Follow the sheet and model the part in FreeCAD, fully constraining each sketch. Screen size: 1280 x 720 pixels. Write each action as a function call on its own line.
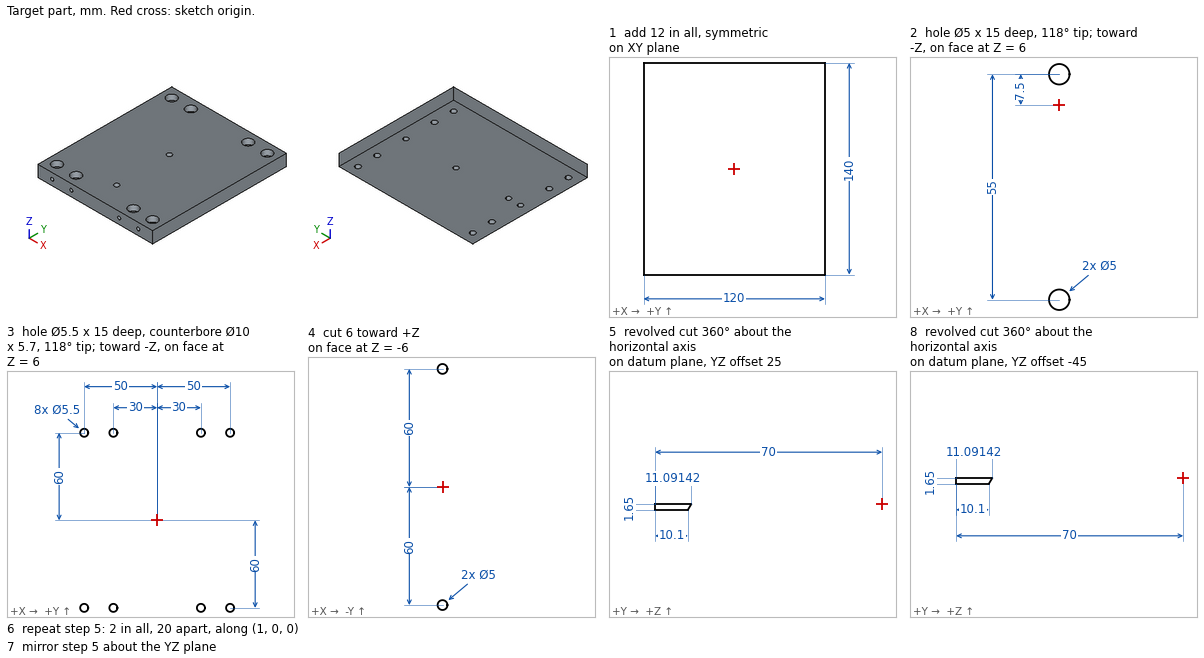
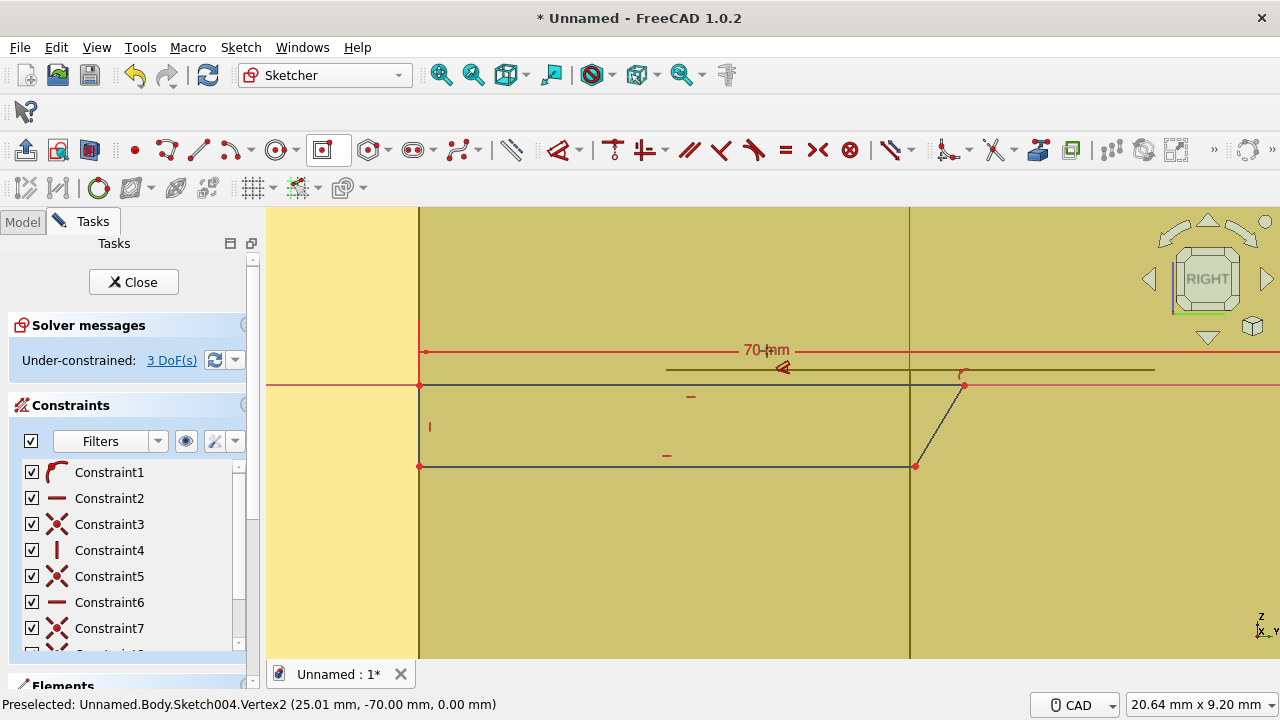
click(419, 410)
click(385, 426)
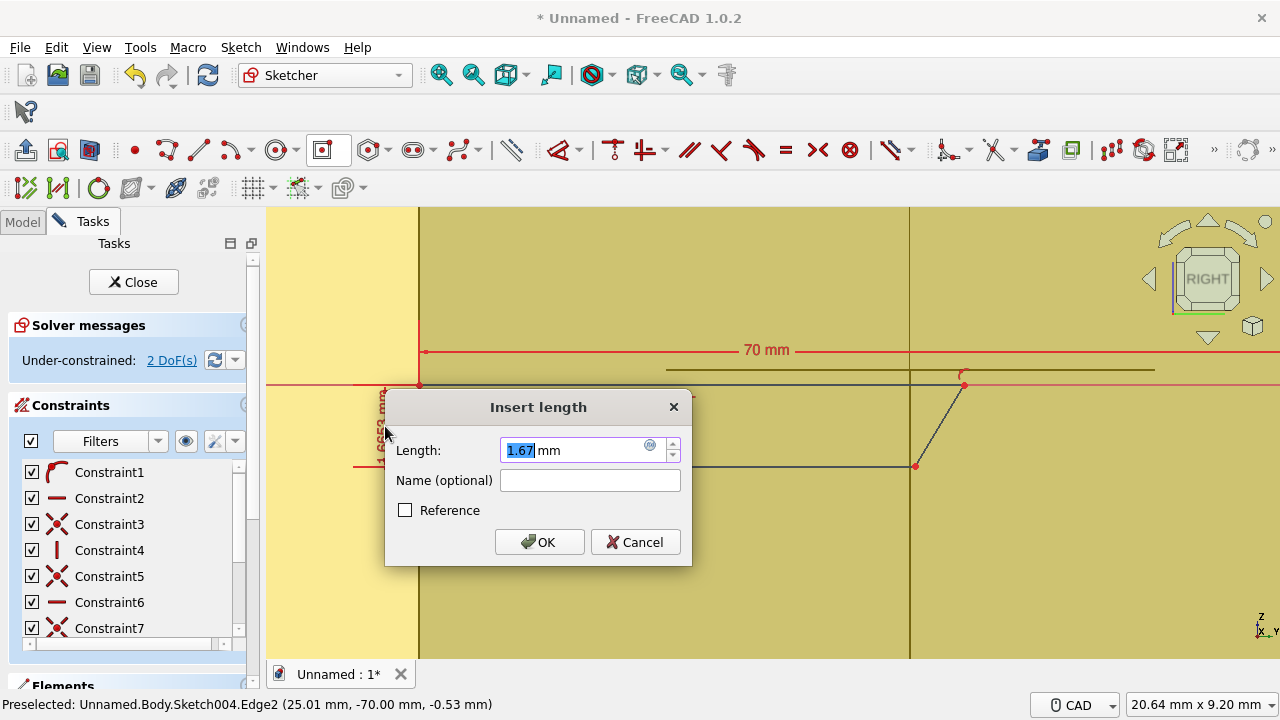
text(1.65)
key(Return)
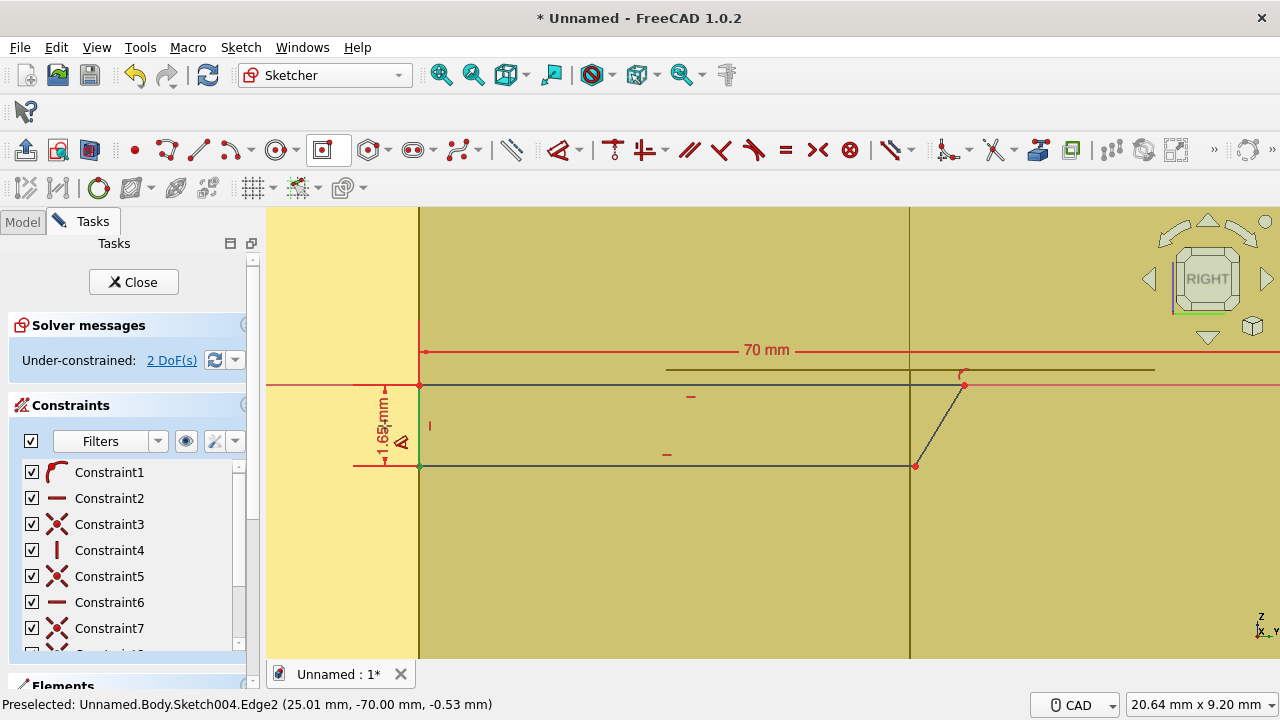
click(568, 466)
click(667, 500)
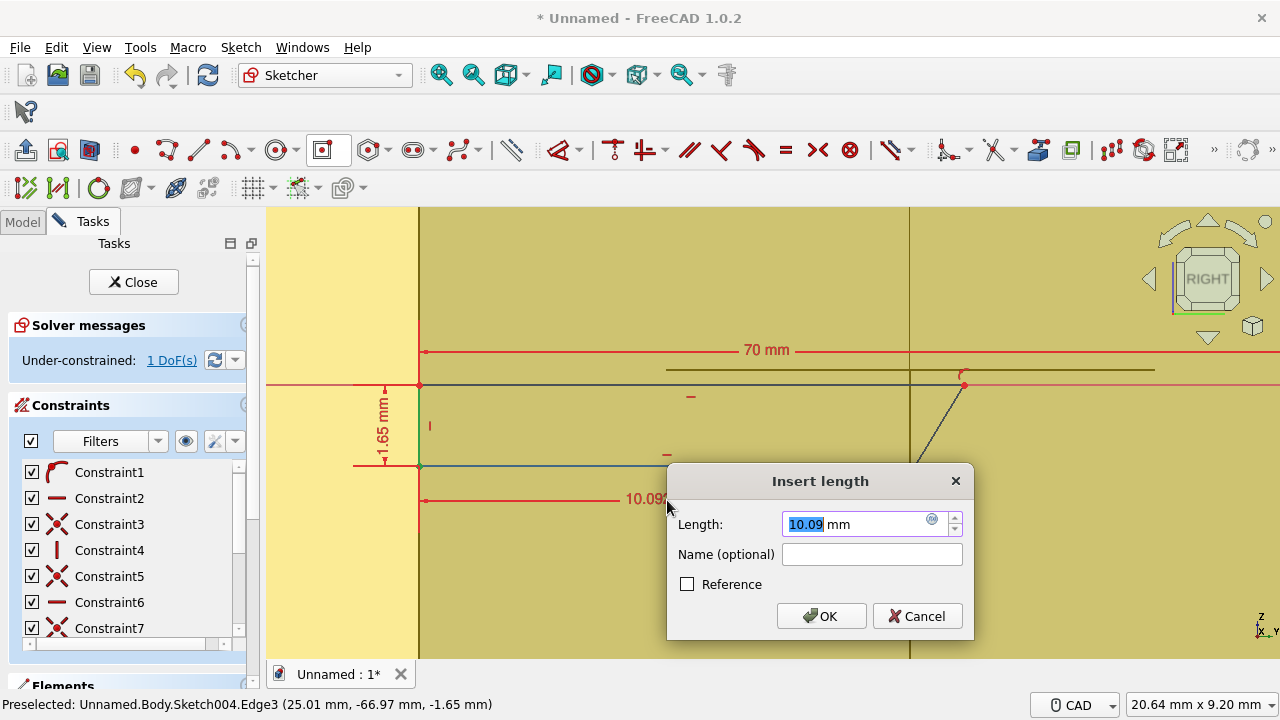
text(10.1)
key(Return)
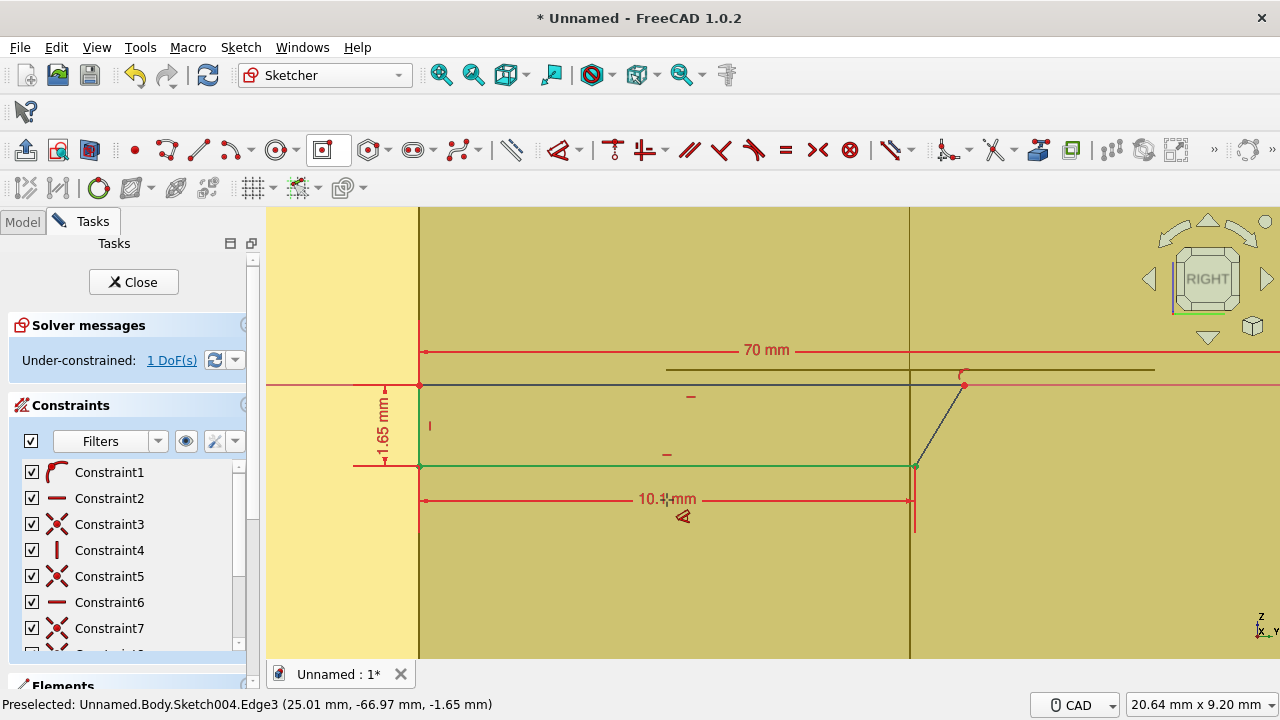
click(801, 385)
click(692, 351)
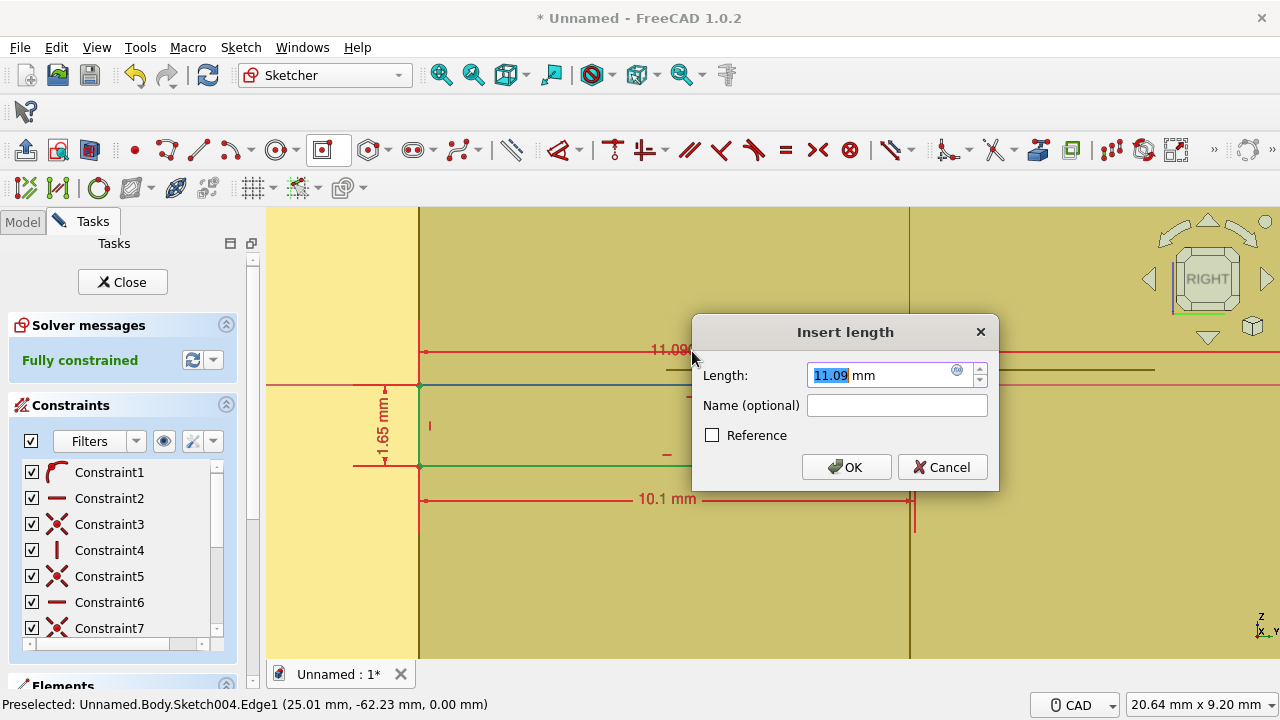
text(11.09142)
key(Return)
key(Escape)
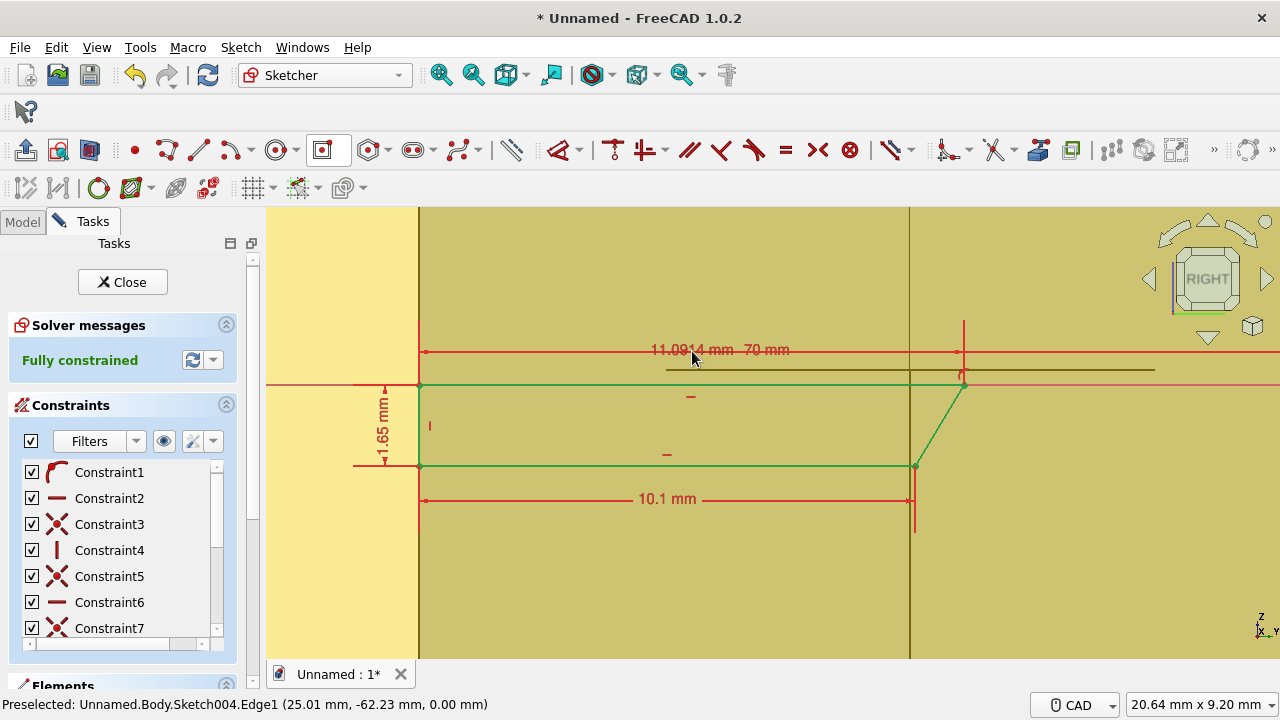
click(123, 282)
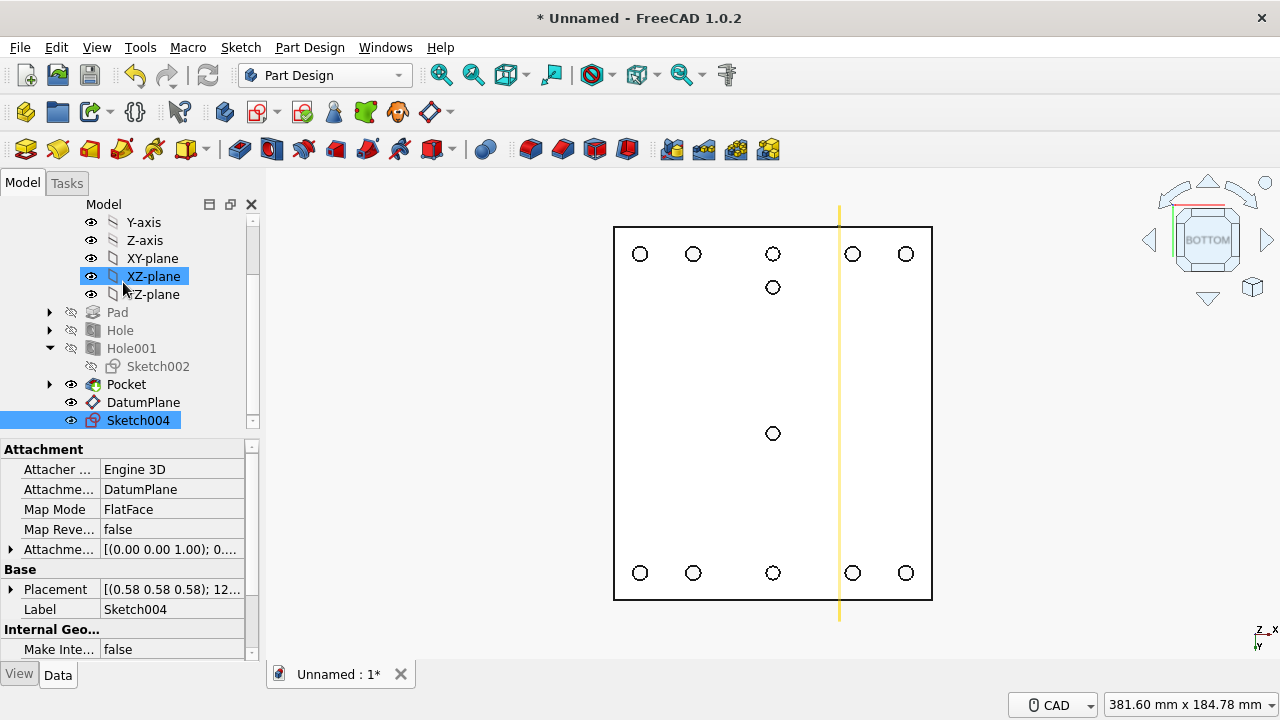
click(304, 150)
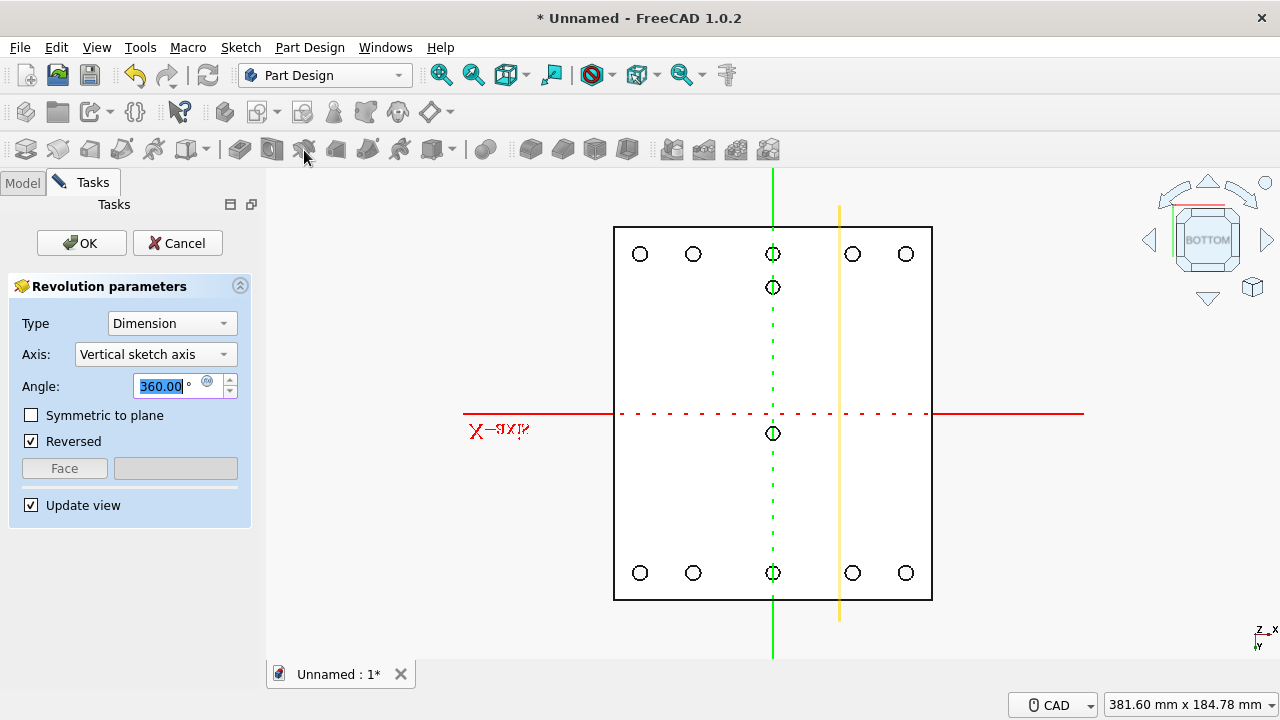
click(156, 354)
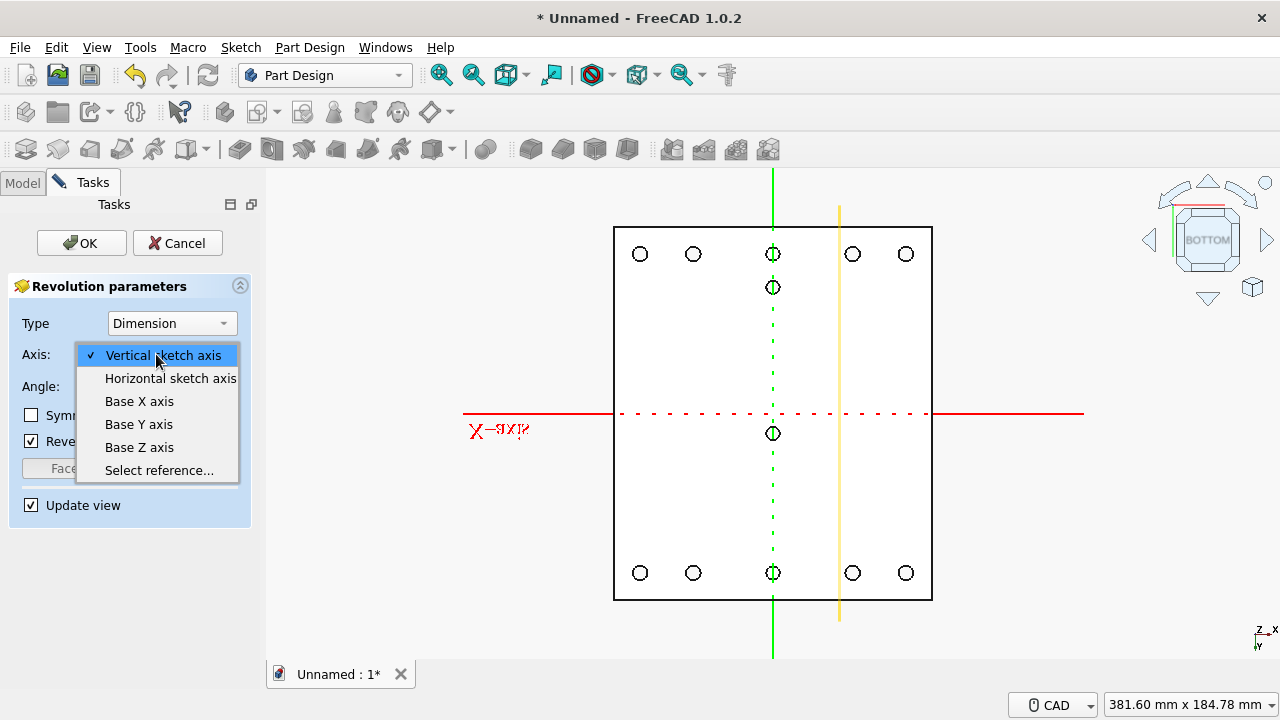
click(156, 378)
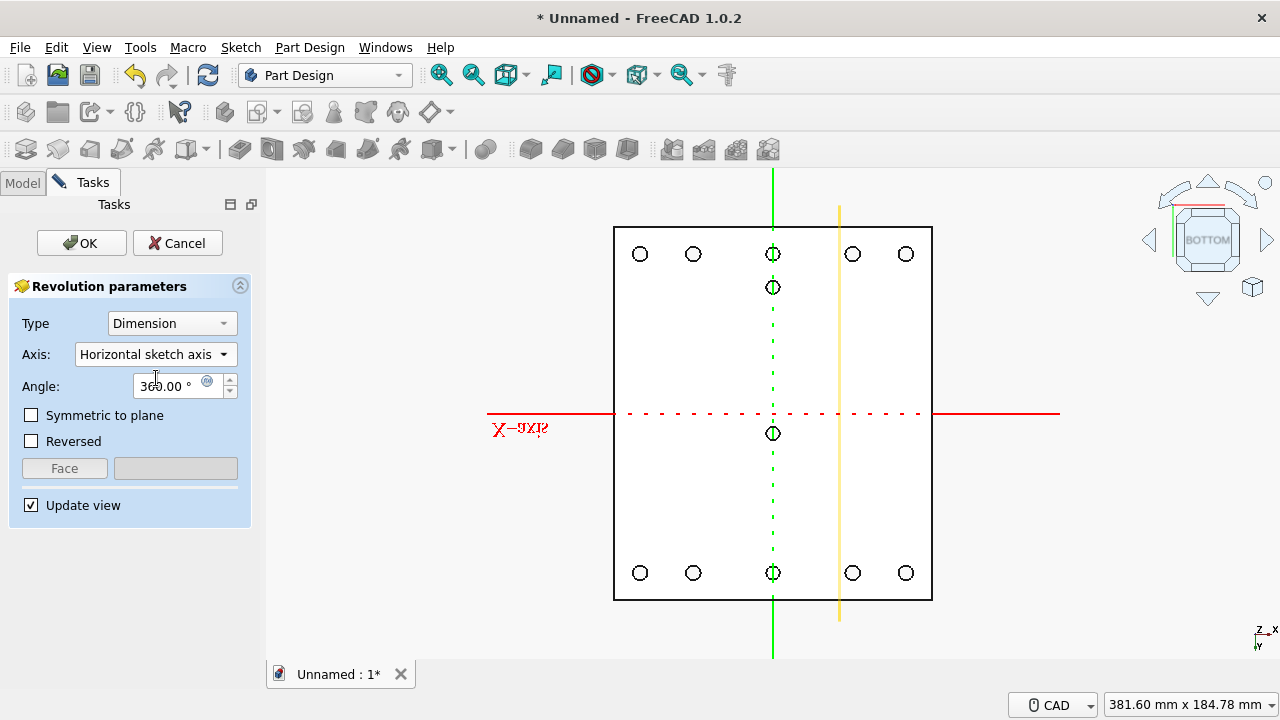
click(82, 243)